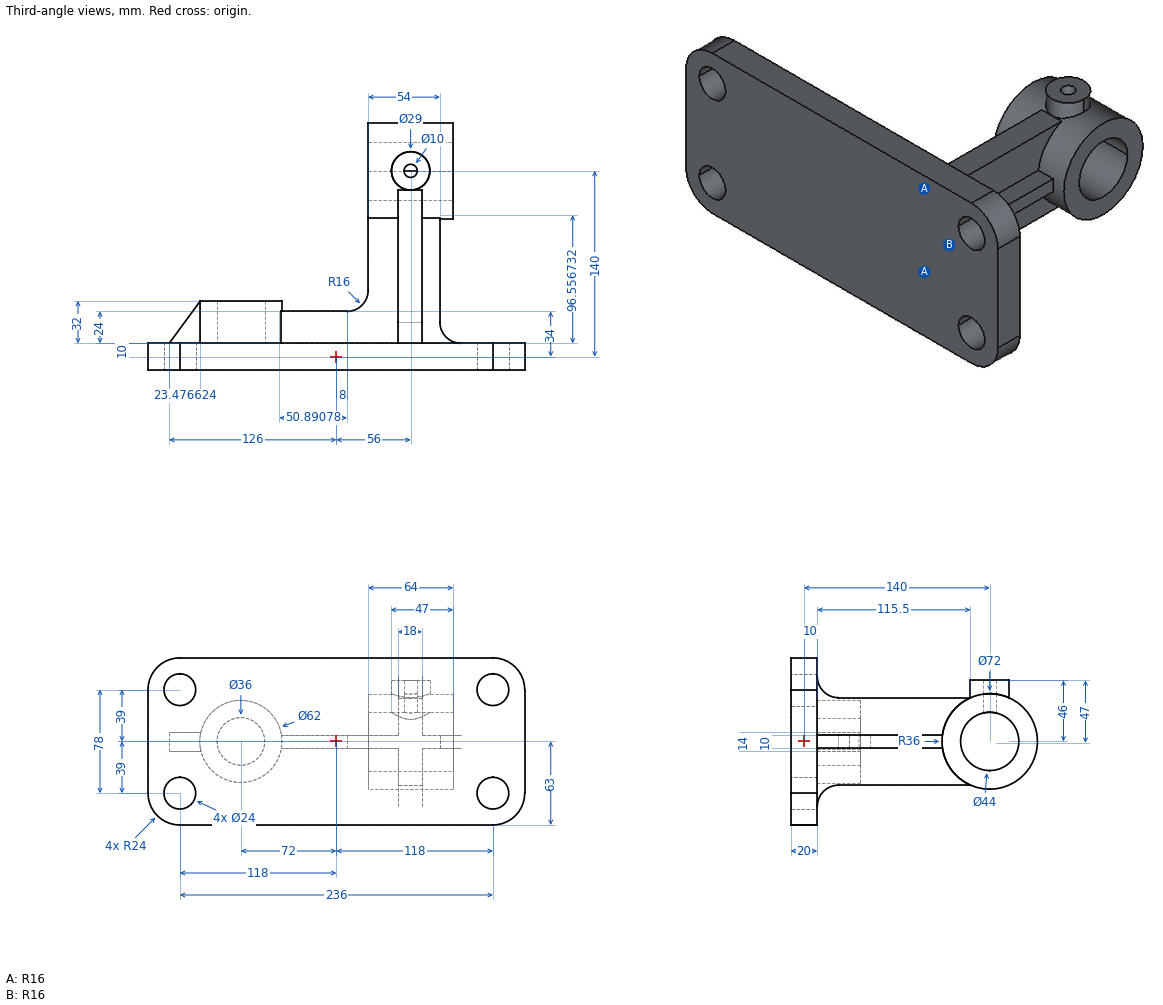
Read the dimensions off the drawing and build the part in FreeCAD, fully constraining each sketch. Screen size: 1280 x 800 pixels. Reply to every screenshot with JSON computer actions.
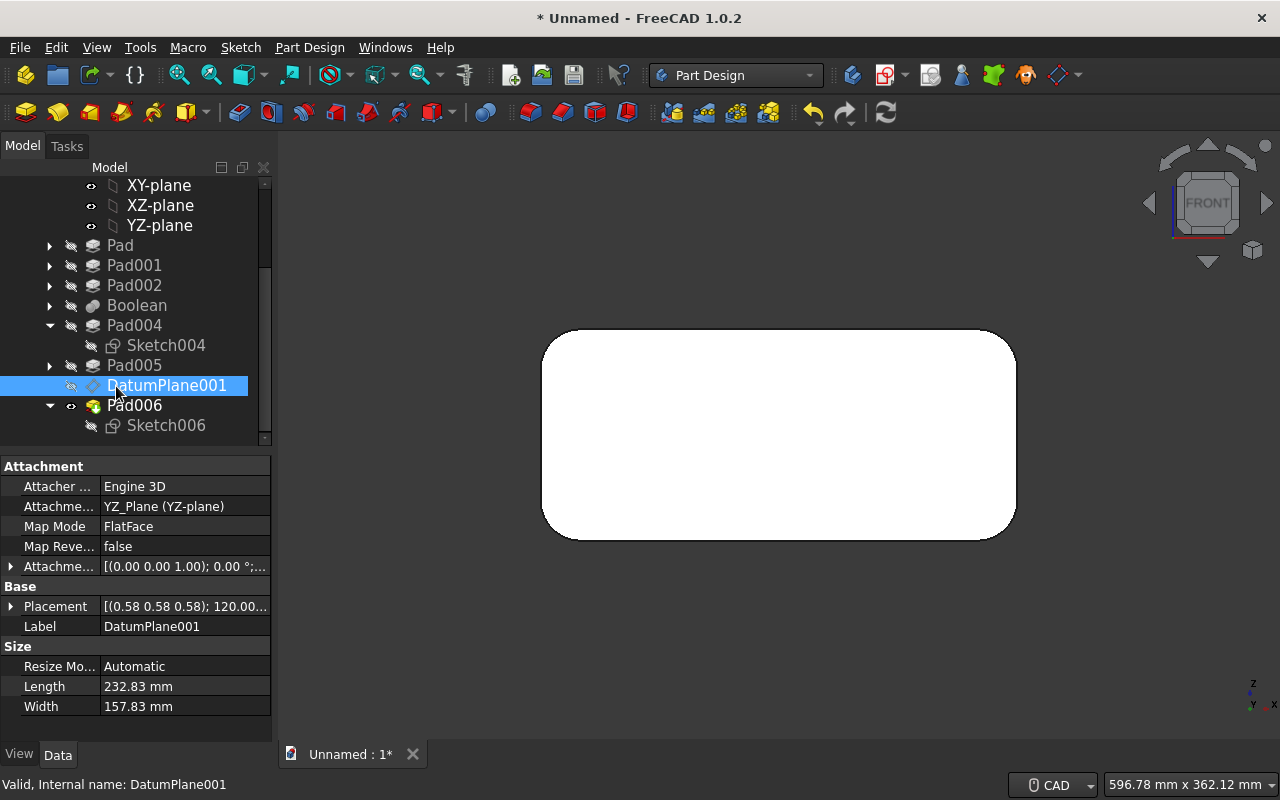
{"action": "key", "text": "3"}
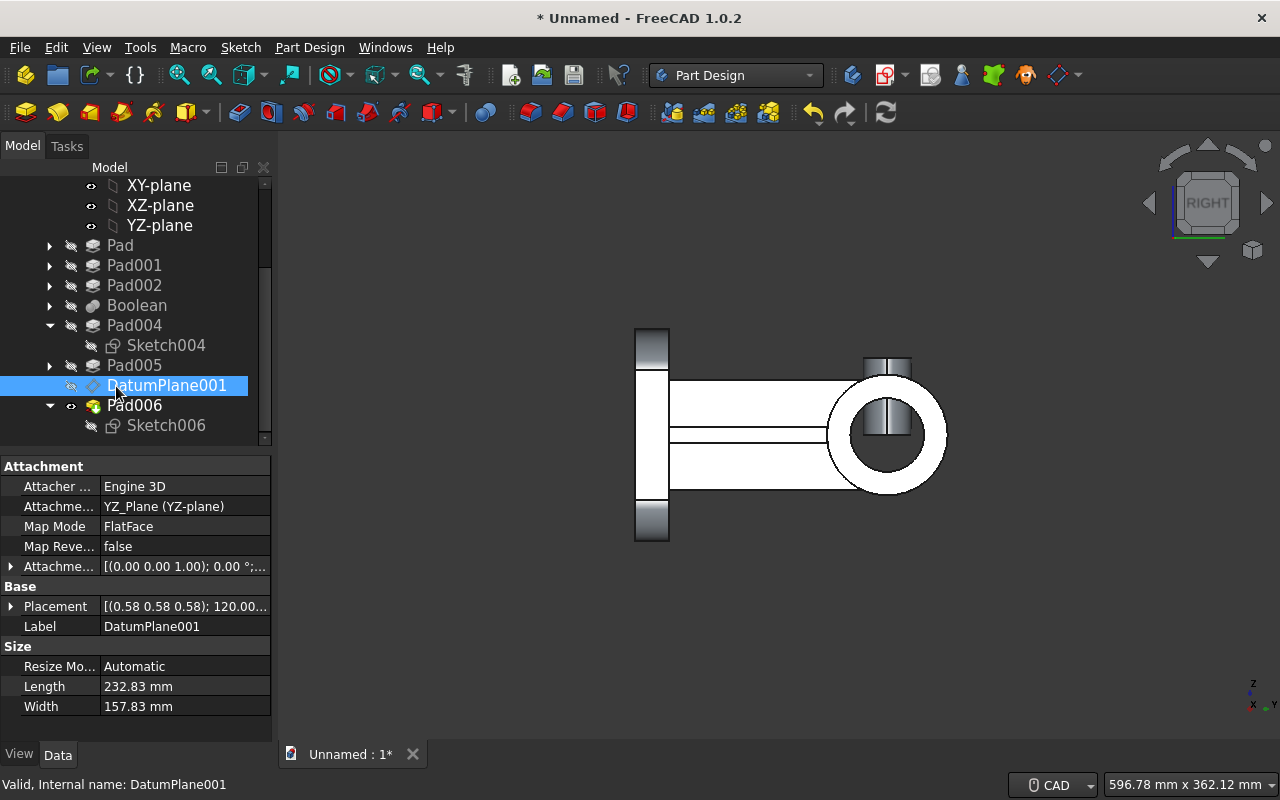
{"action": "left_click", "coordinate": [180, 76]}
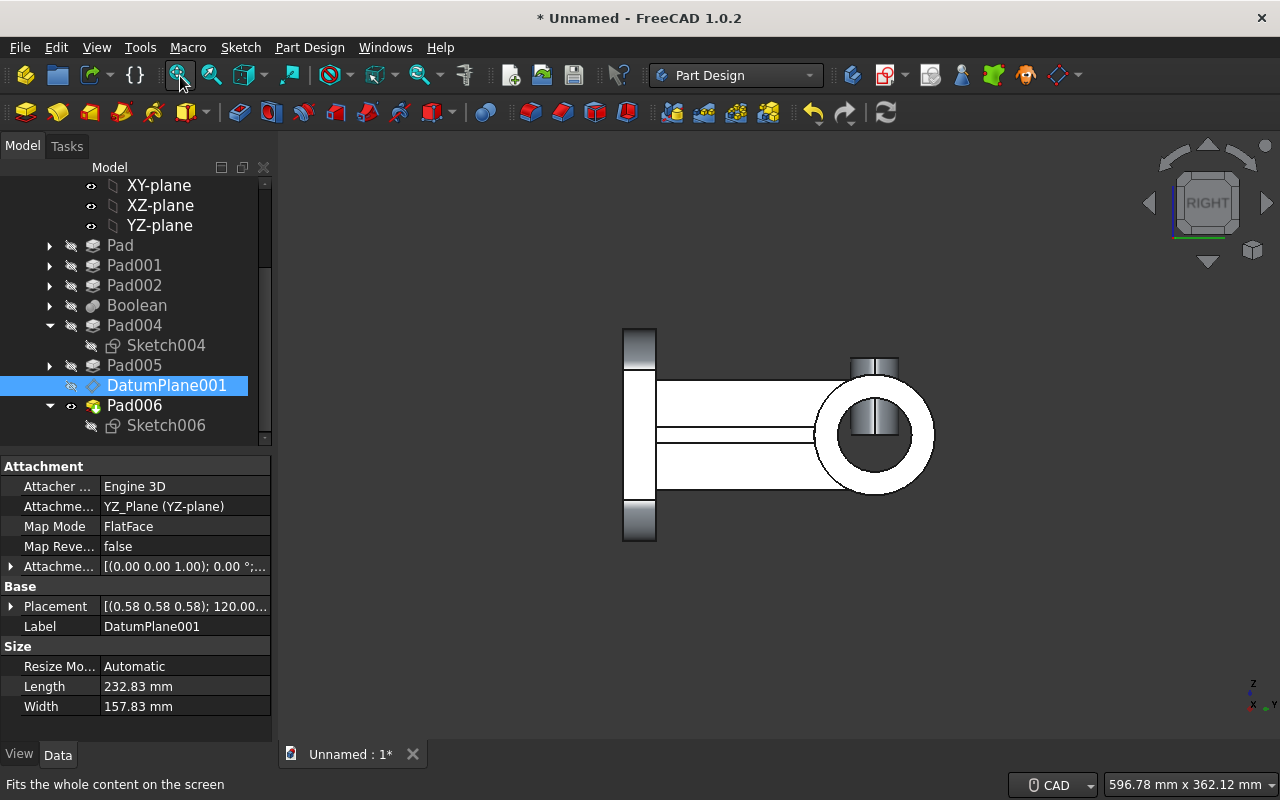
{"action": "key", "text": "5"}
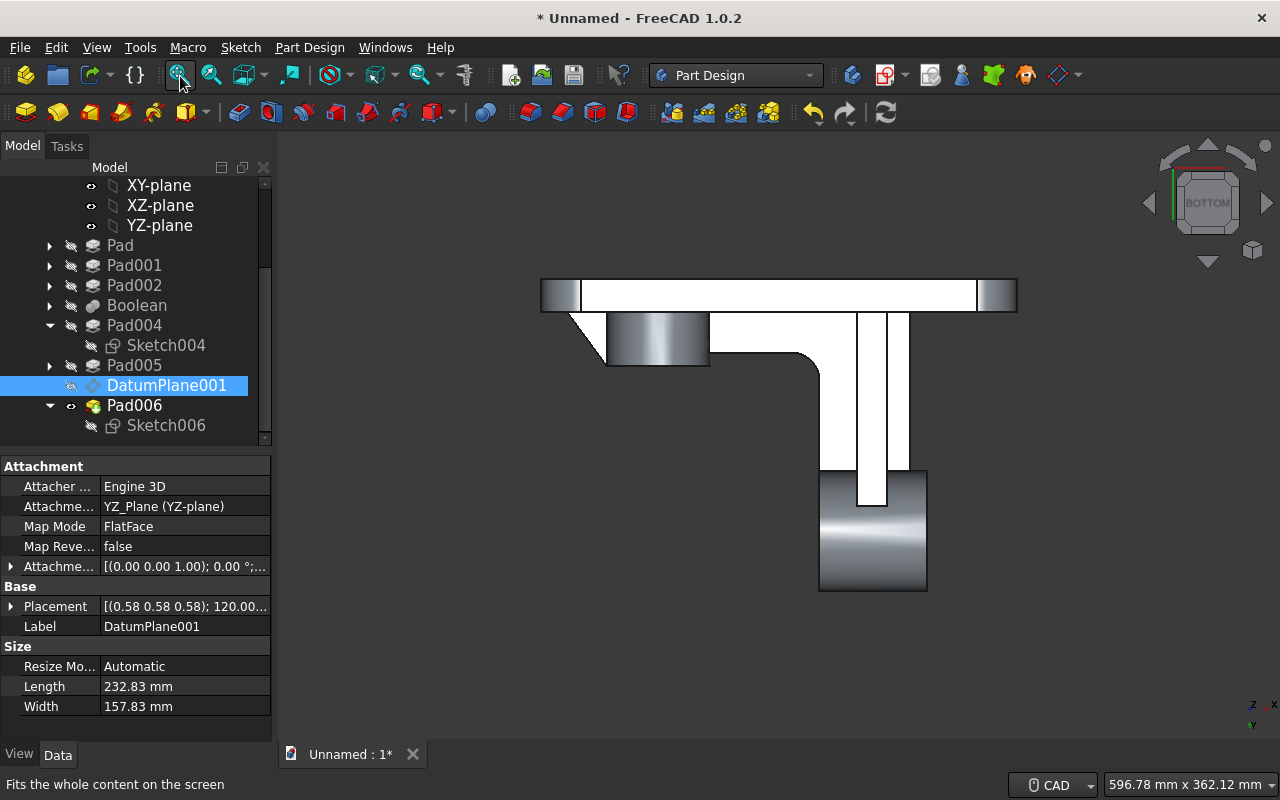
{"action": "key", "text": "4"}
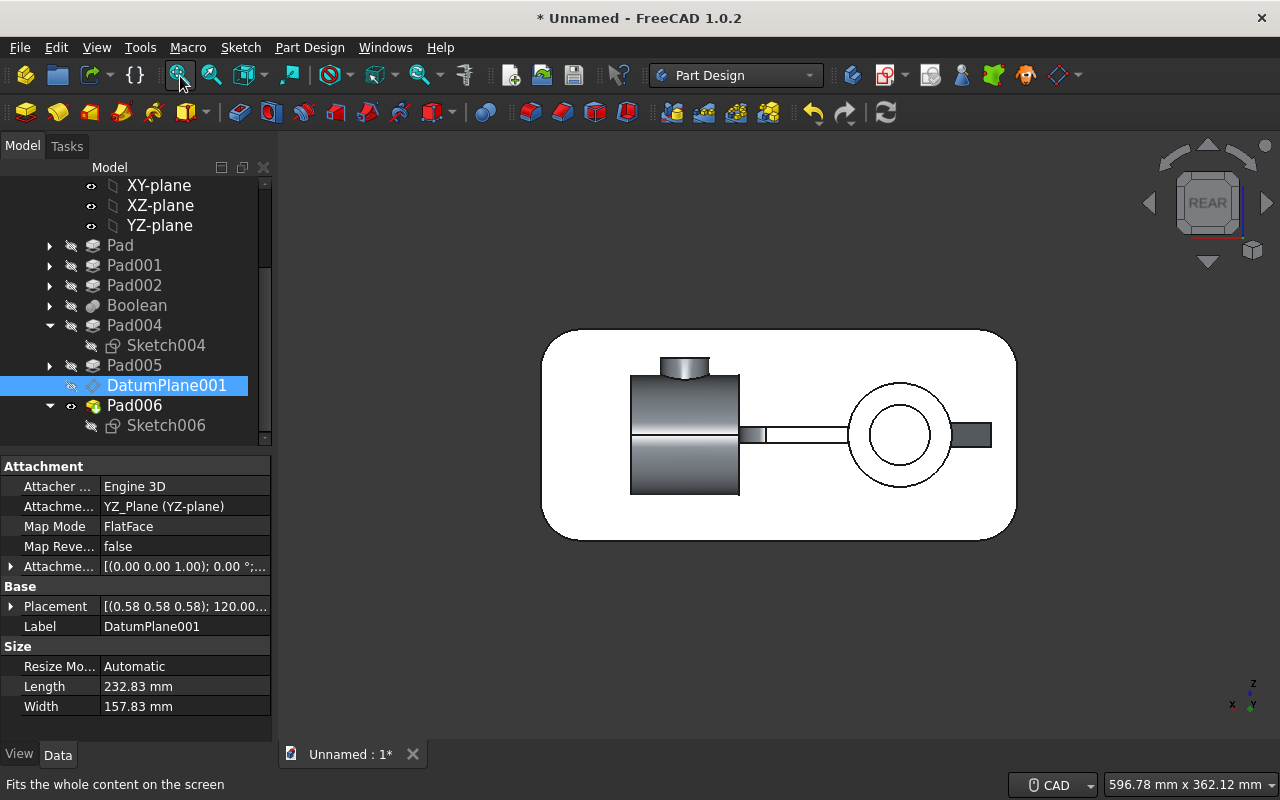
{"action": "key", "text": "6"}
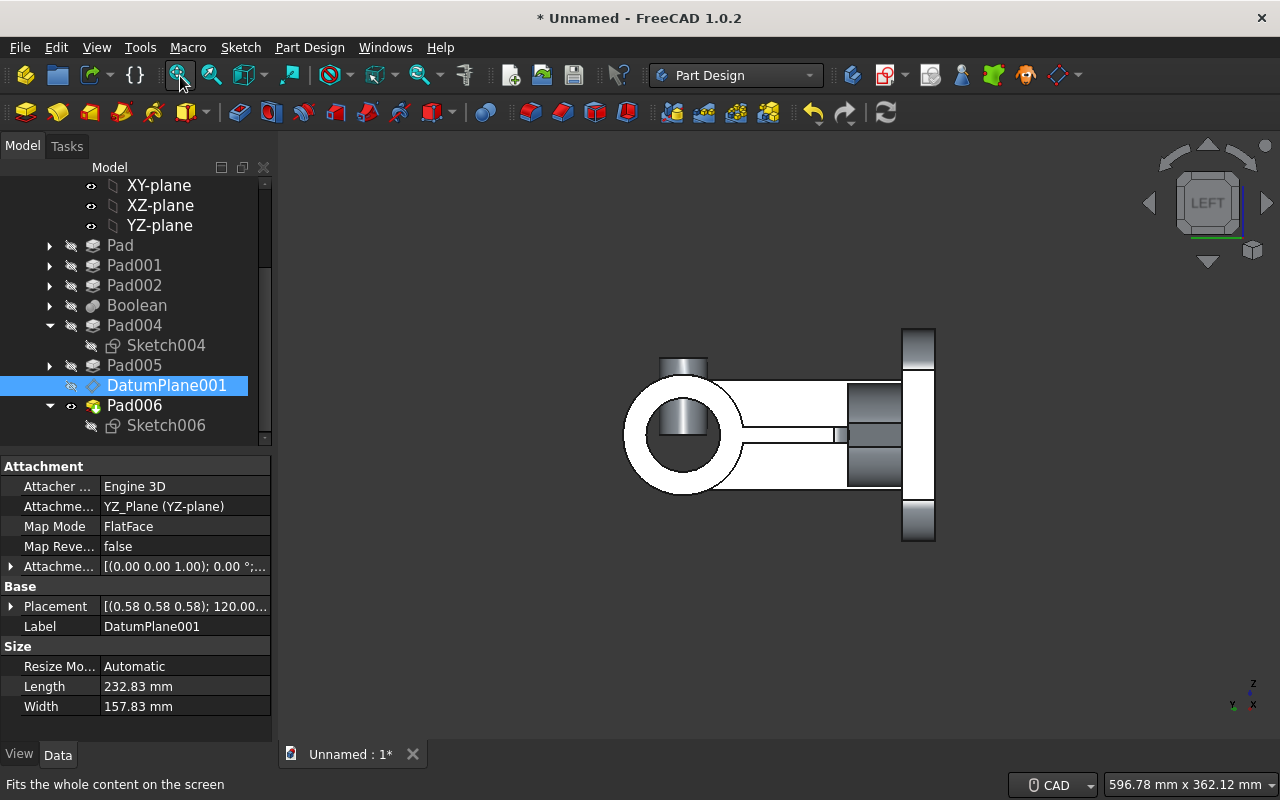
{"action": "left_click", "coordinate": [180, 76]}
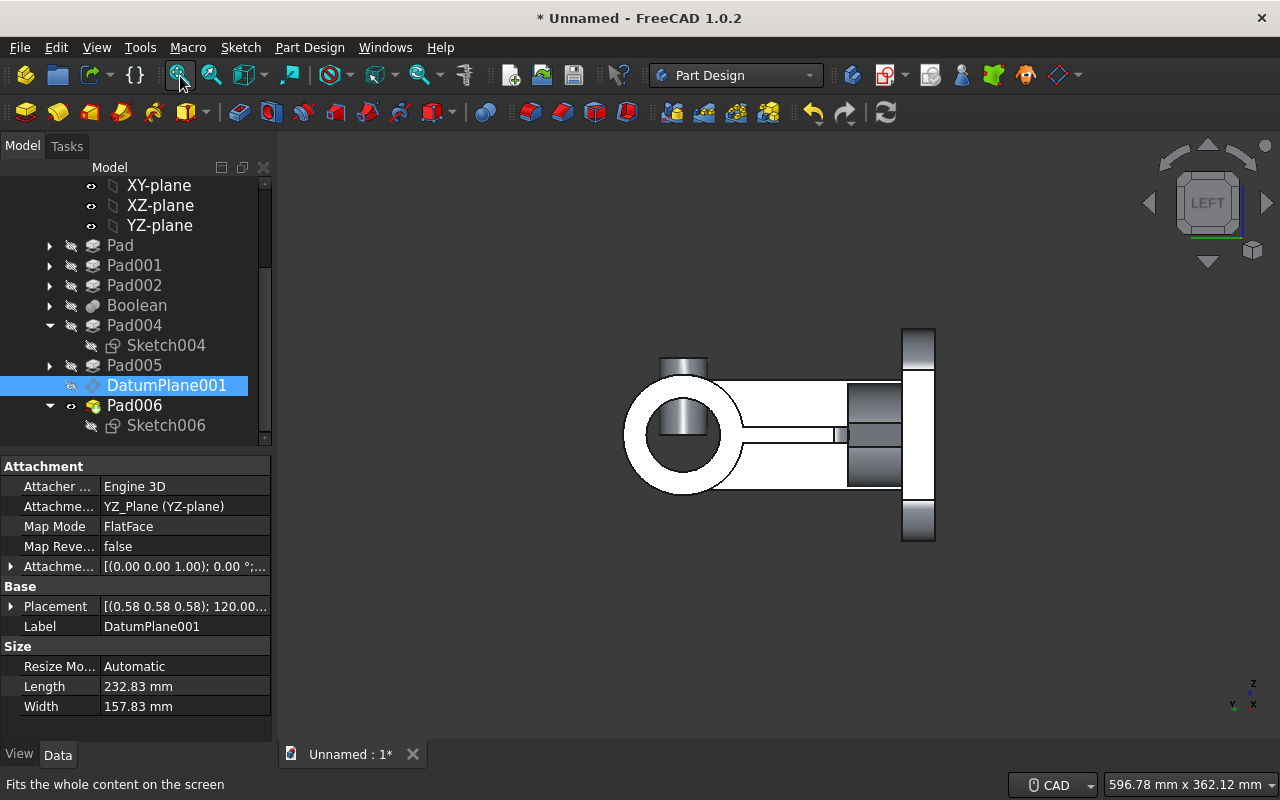
{"action": "key", "text": "v 3"}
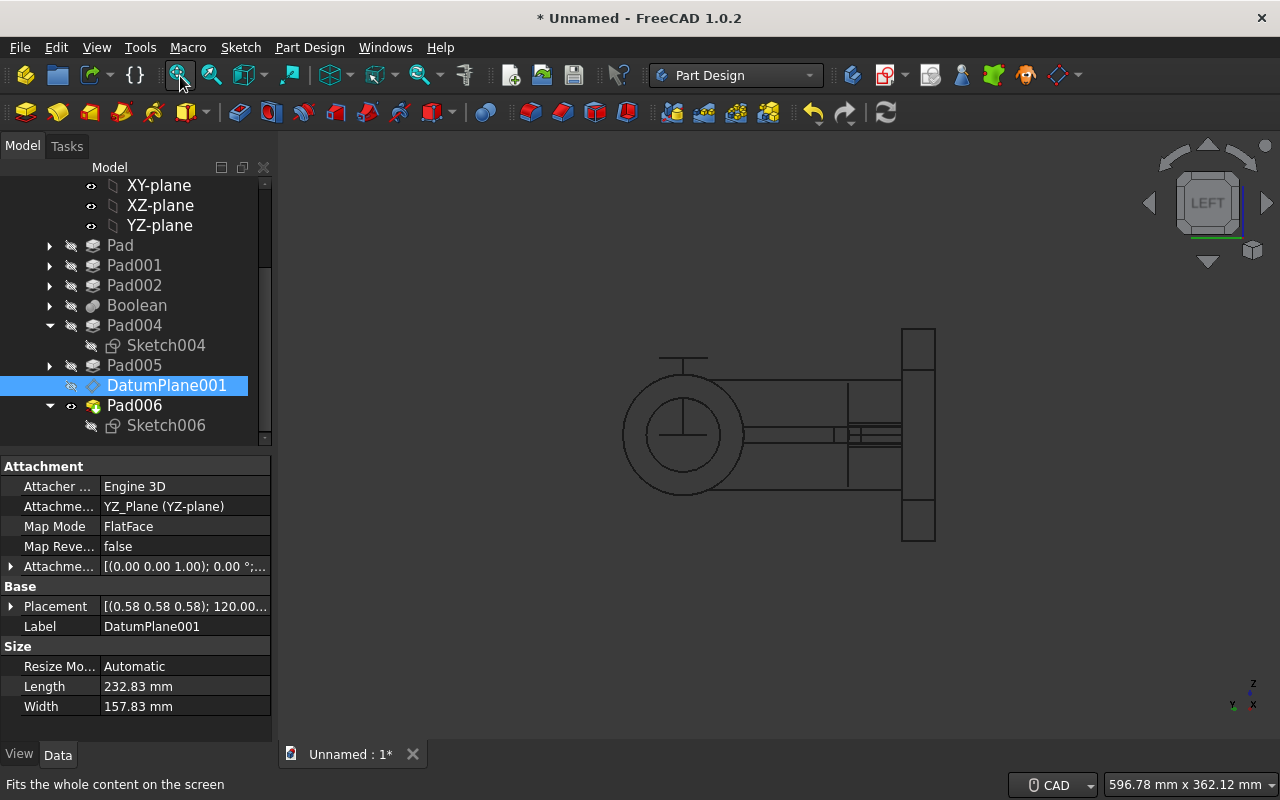
{"action": "key", "text": "0"}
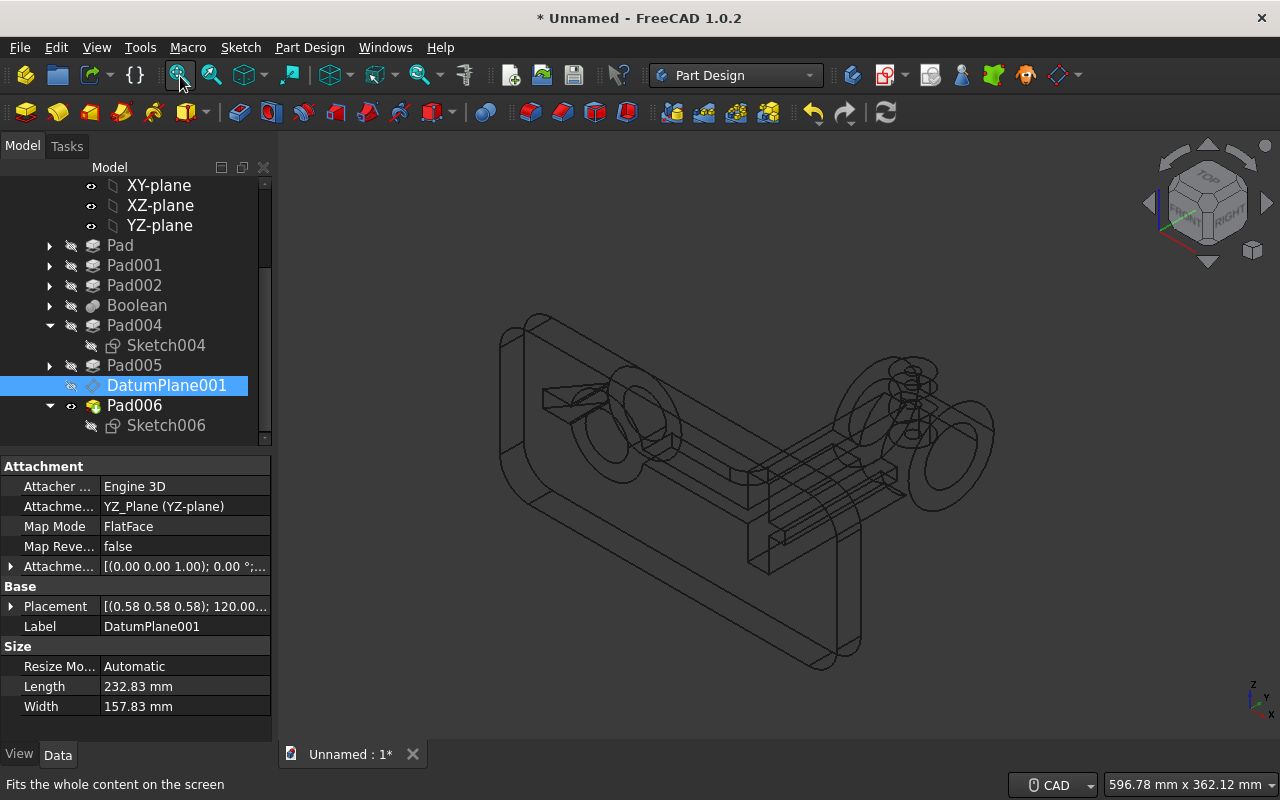
{"action": "left_click", "coordinate": [758, 567]}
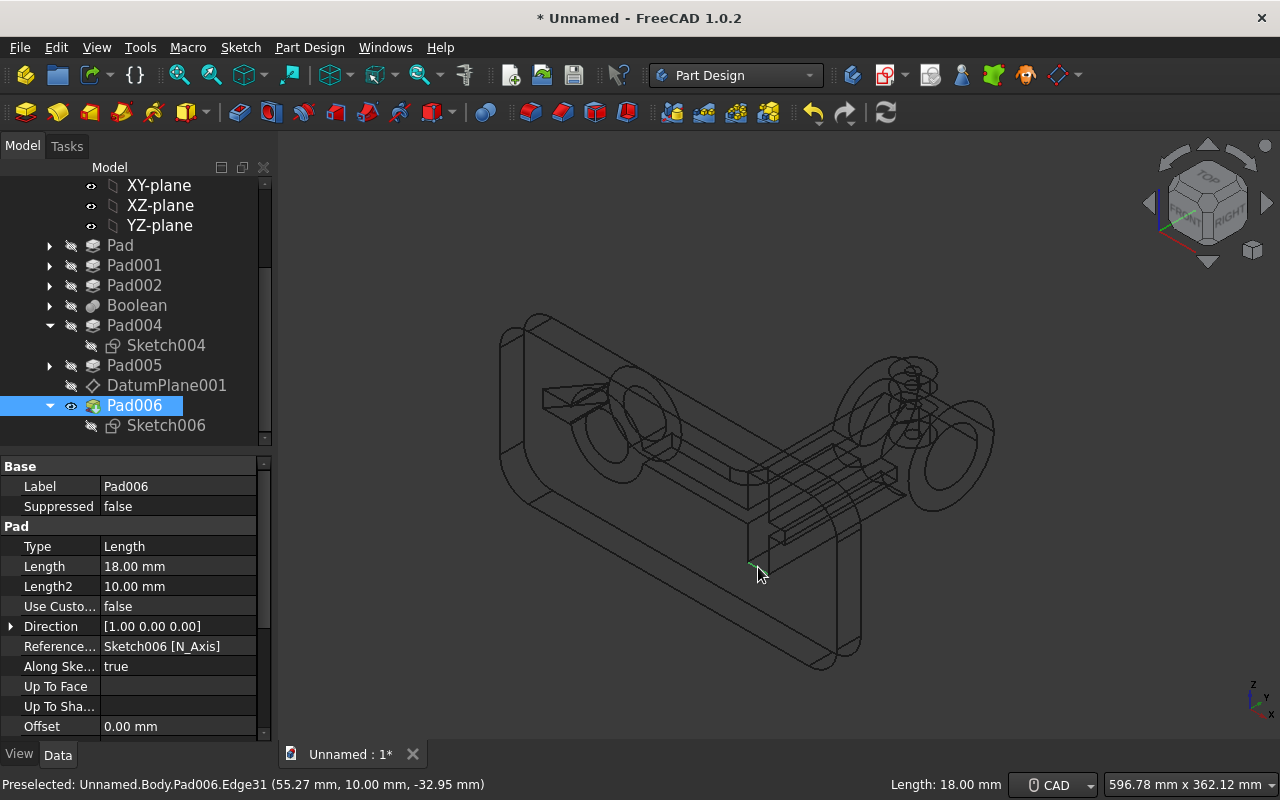
{"action": "left_click", "coordinate": [758, 477], "text": "ctrl"}